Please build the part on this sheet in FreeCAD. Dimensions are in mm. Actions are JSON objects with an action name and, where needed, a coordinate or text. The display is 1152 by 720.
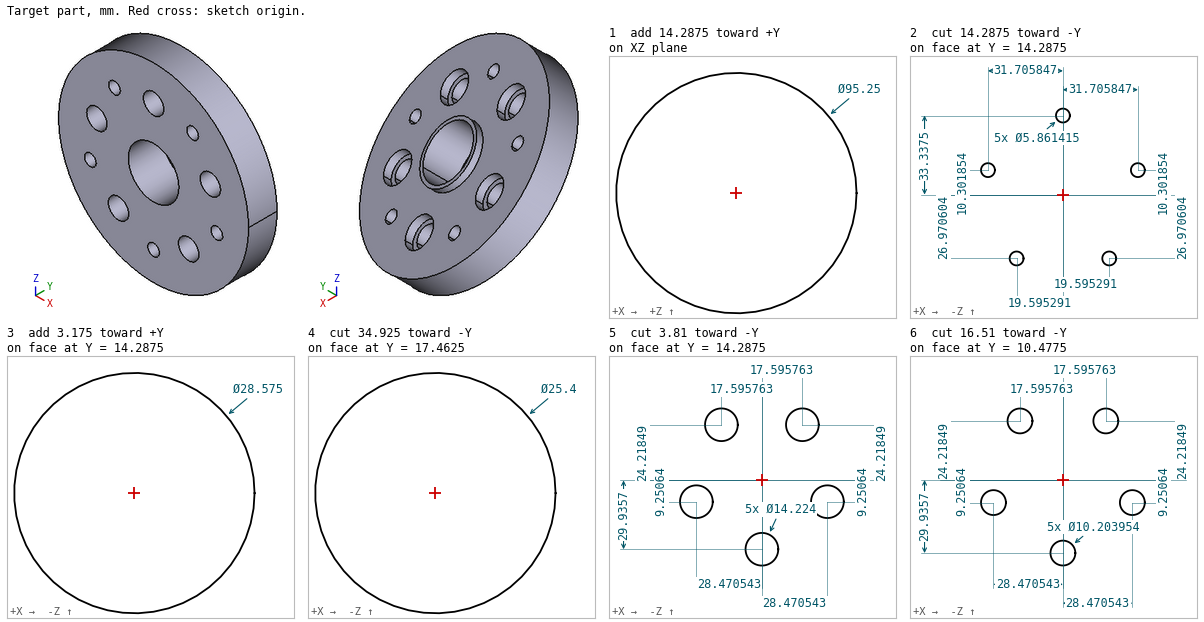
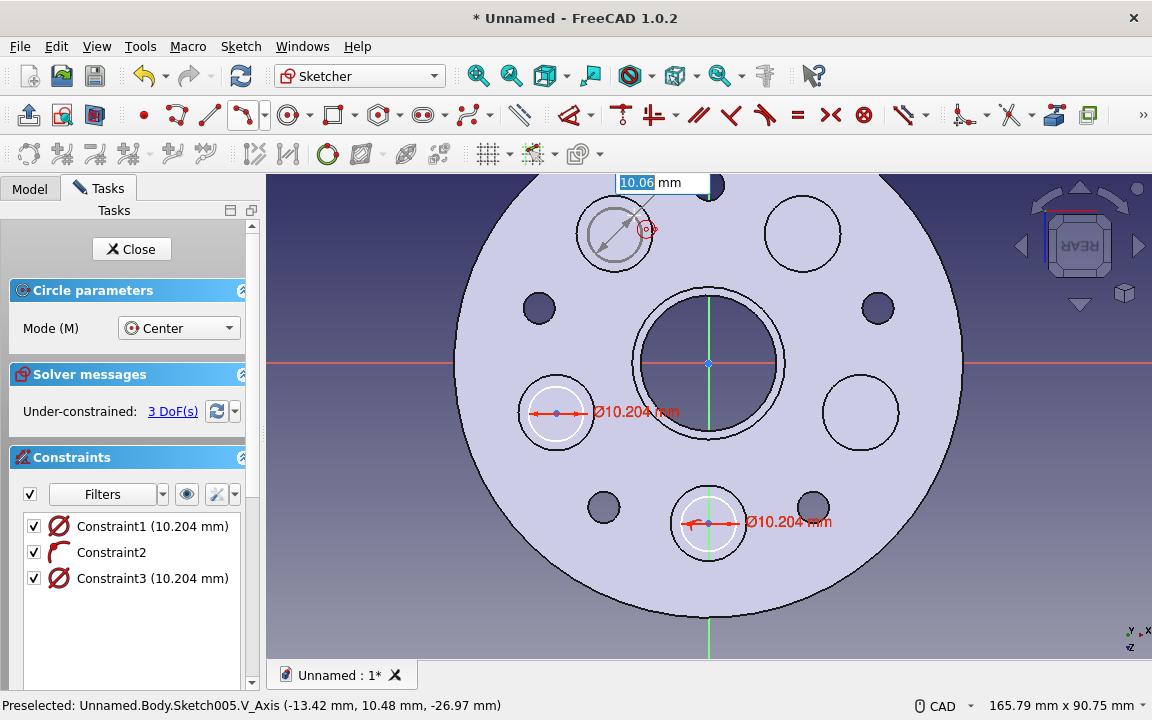
{"action": "type", "text": "10.203954"}
{"action": "key", "text": "Return"}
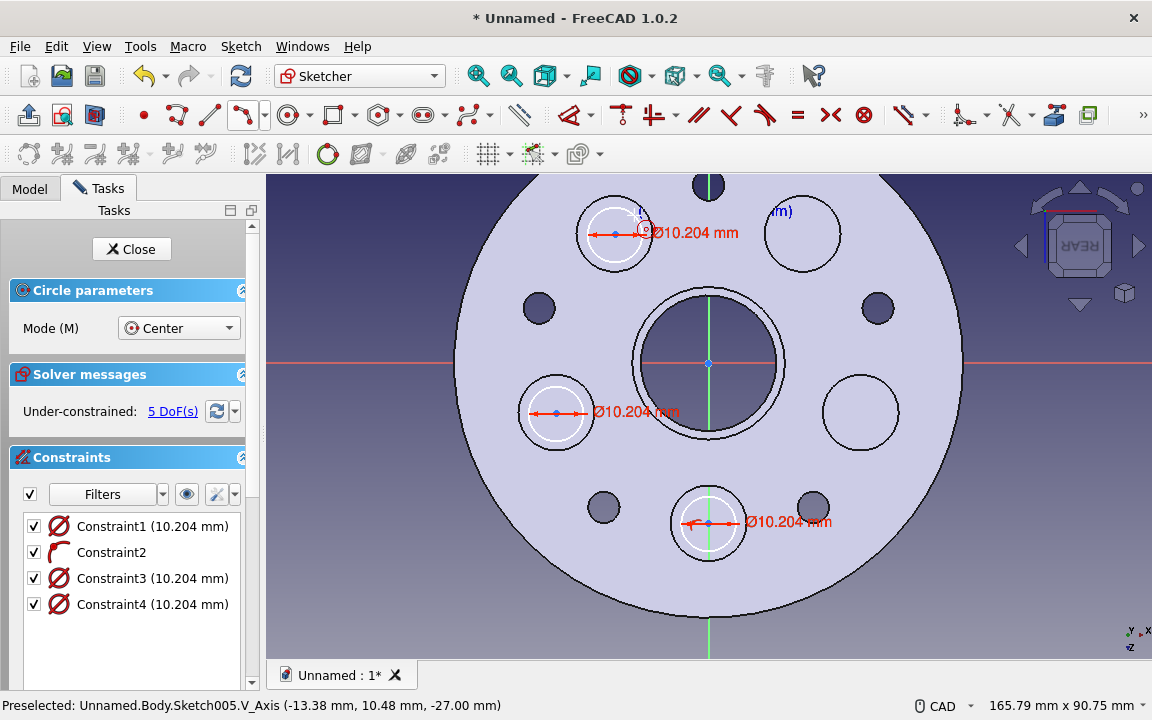
{"action": "left_click", "coordinate": [803, 234]}
{"action": "mouse_move", "coordinate": [822, 215]}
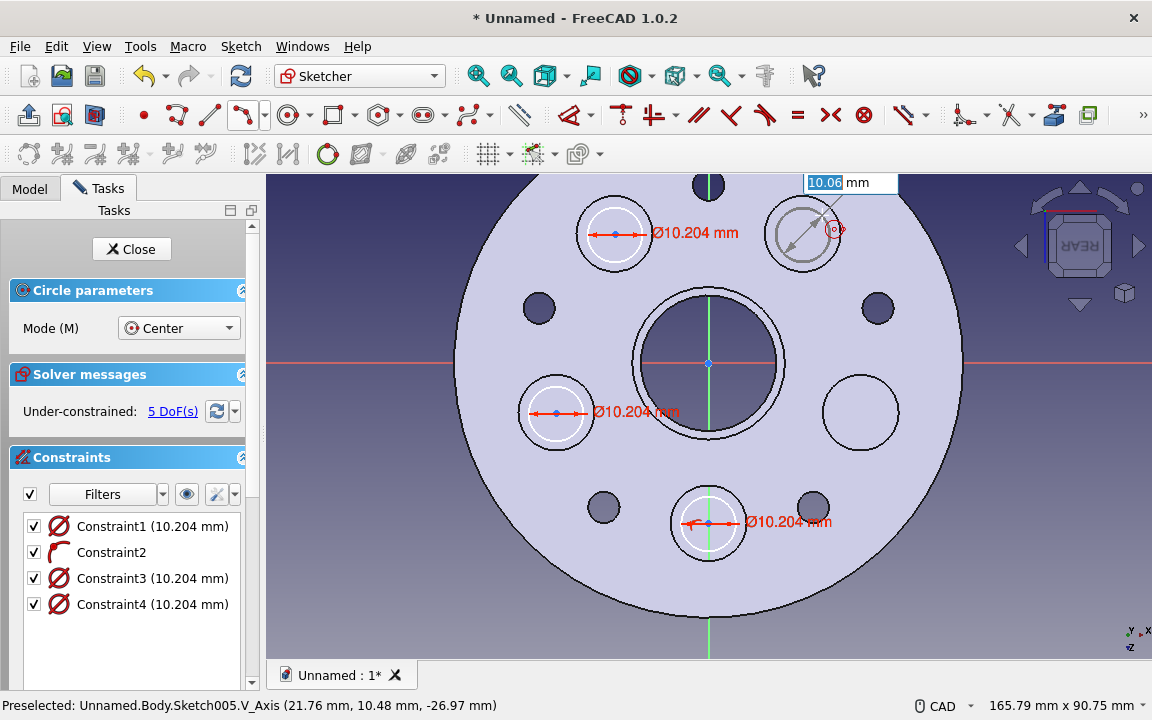
{"action": "type", "text": "10.203954"}
{"action": "key", "text": "Return"}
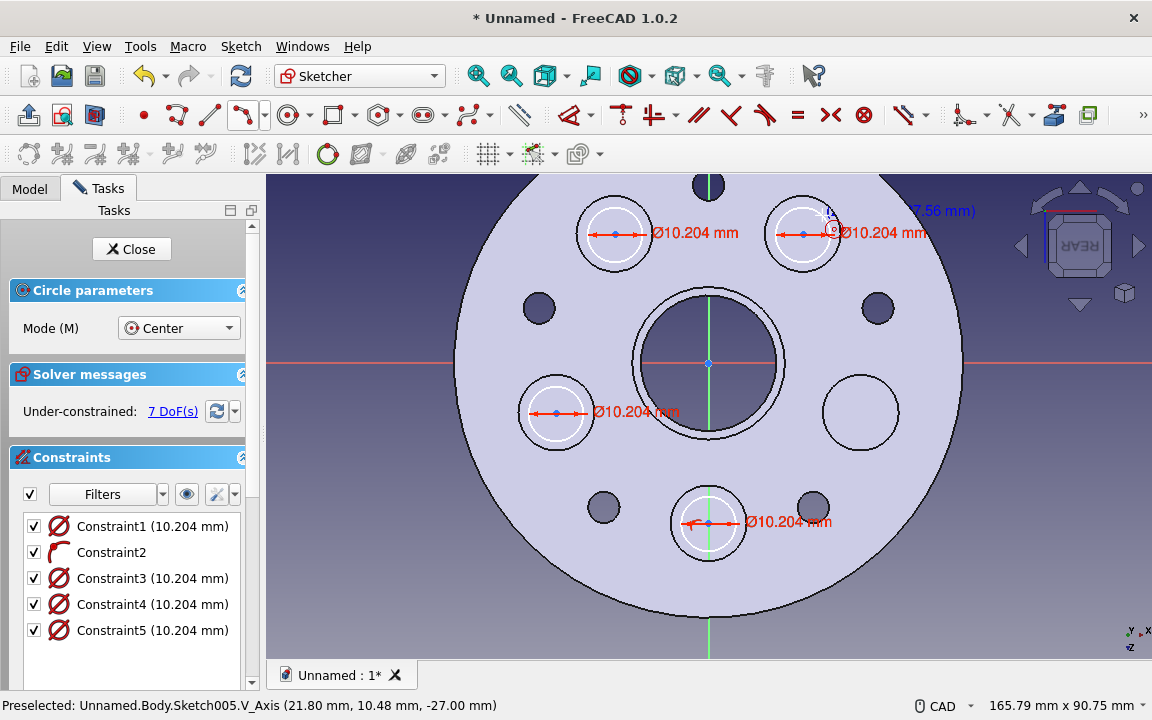
{"action": "left_click", "coordinate": [861, 413]}
{"action": "mouse_move", "coordinate": [880, 393]}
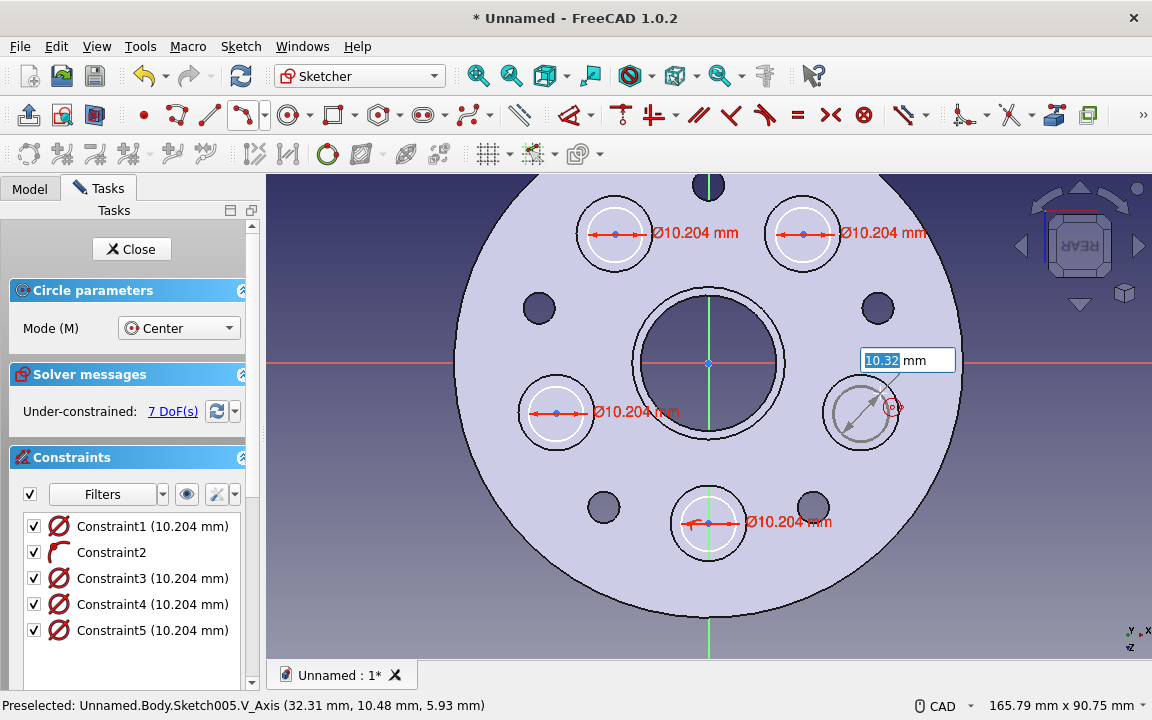
{"action": "type", "text": "10.203954"}
{"action": "key", "text": "Return"}
{"action": "key", "text": "Escape"}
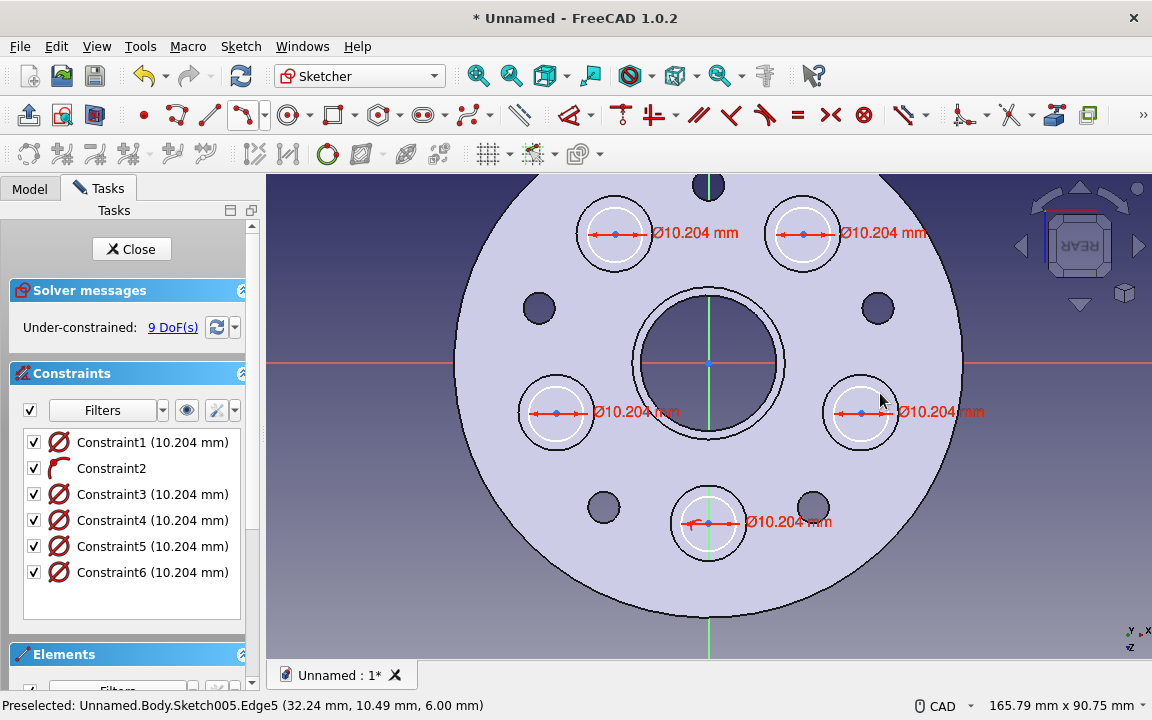
{"action": "left_click", "coordinate": [568, 116]}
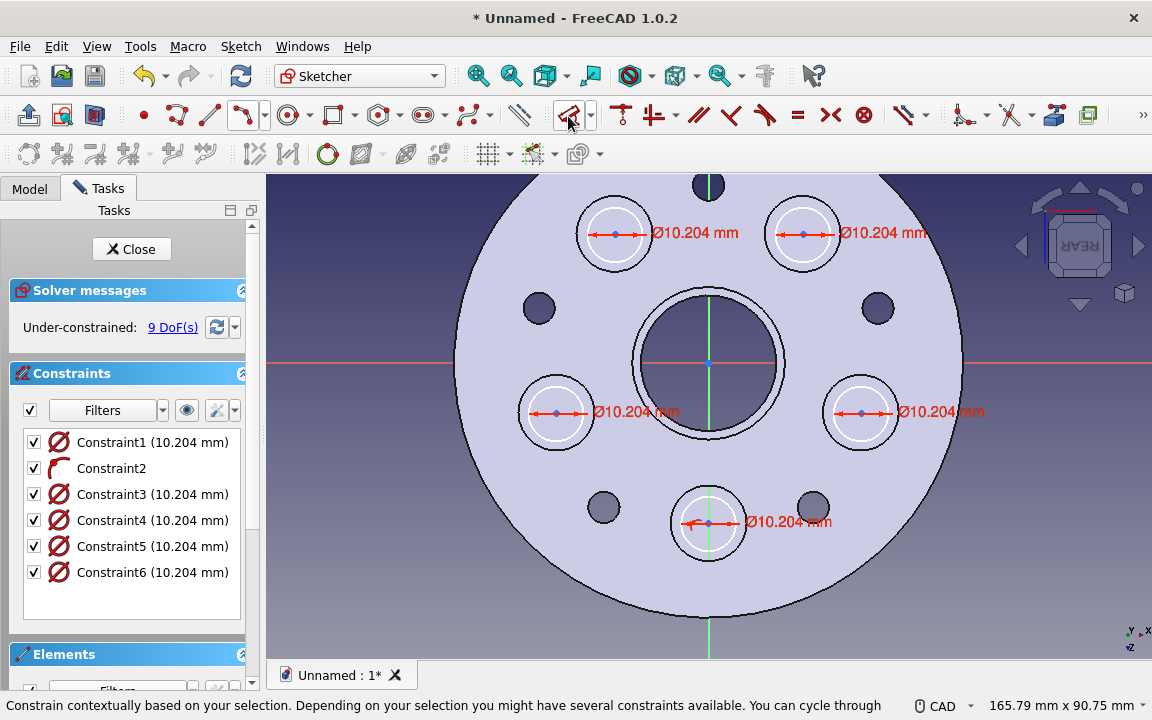
{"action": "left_click", "coordinate": [709, 524]}
{"action": "left_click", "coordinate": [743, 444]}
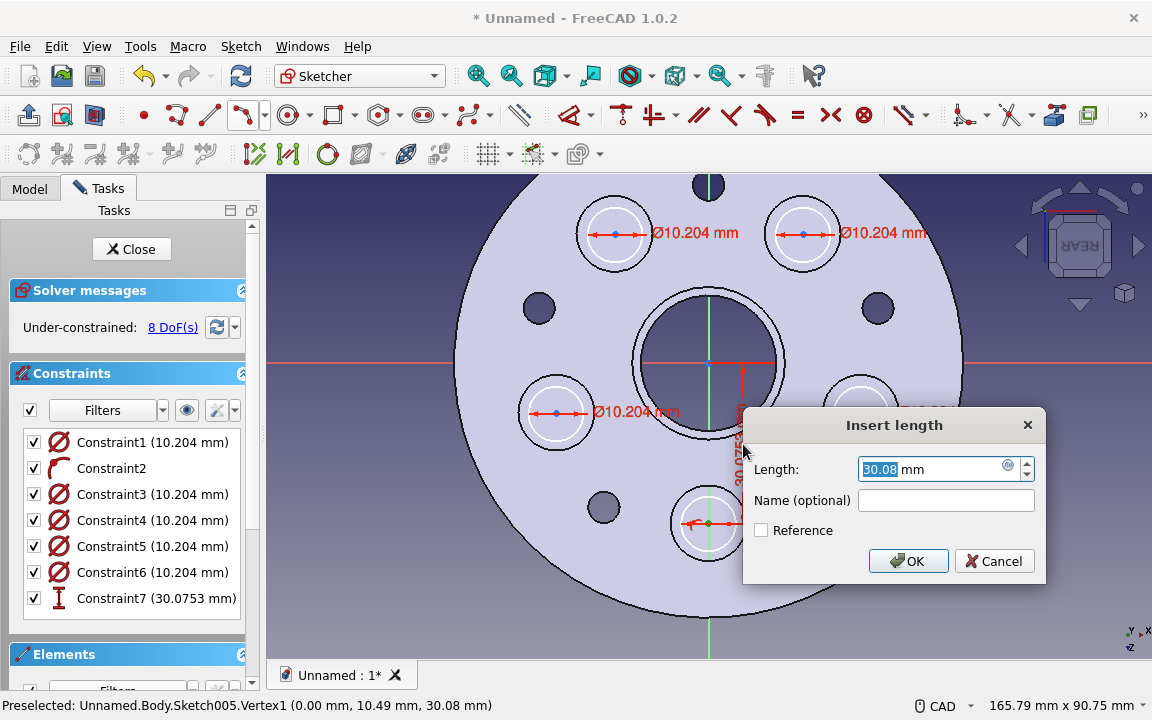
{"action": "type", "text": "29.9357"}
{"action": "key", "text": "Return"}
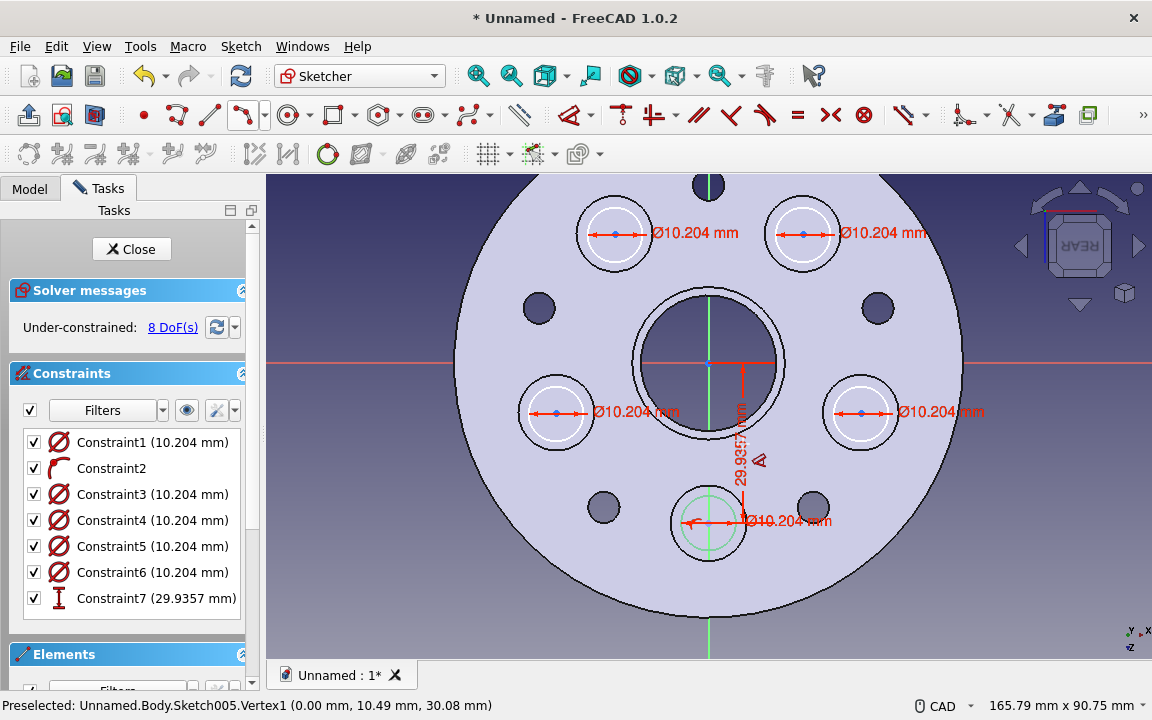
{"action": "left_click", "coordinate": [556, 414]}
{"action": "left_click", "coordinate": [522, 389]}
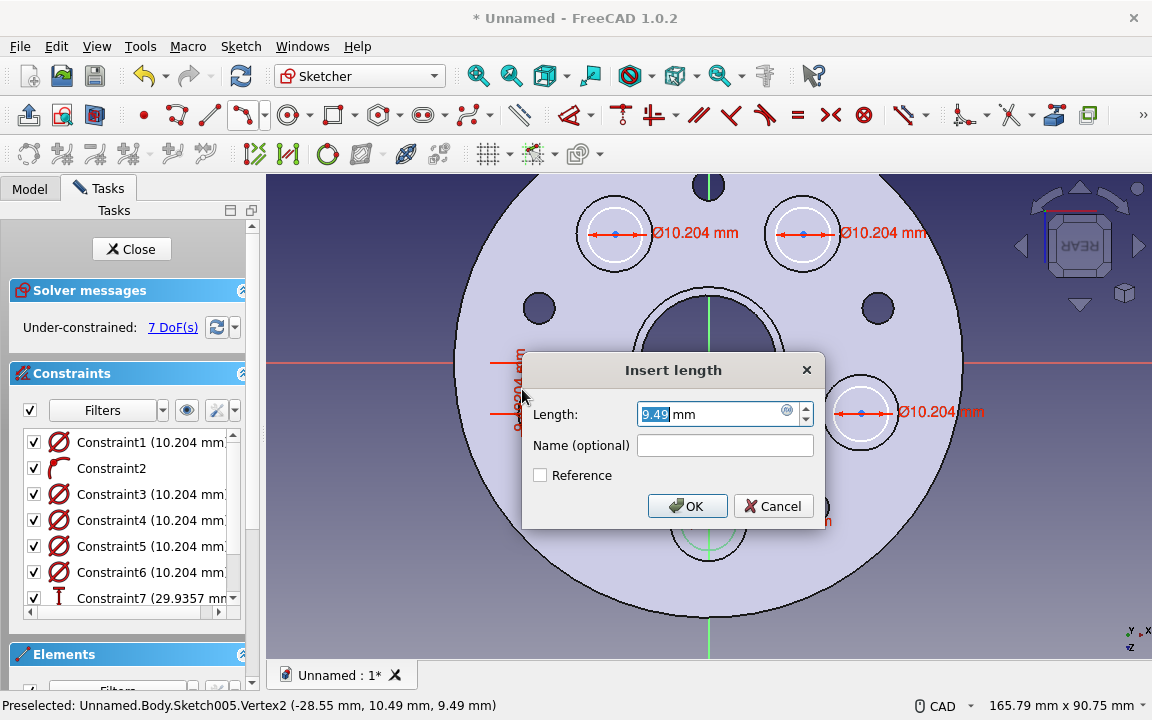
{"action": "type", "text": "9.25064"}
{"action": "key", "text": "Return"}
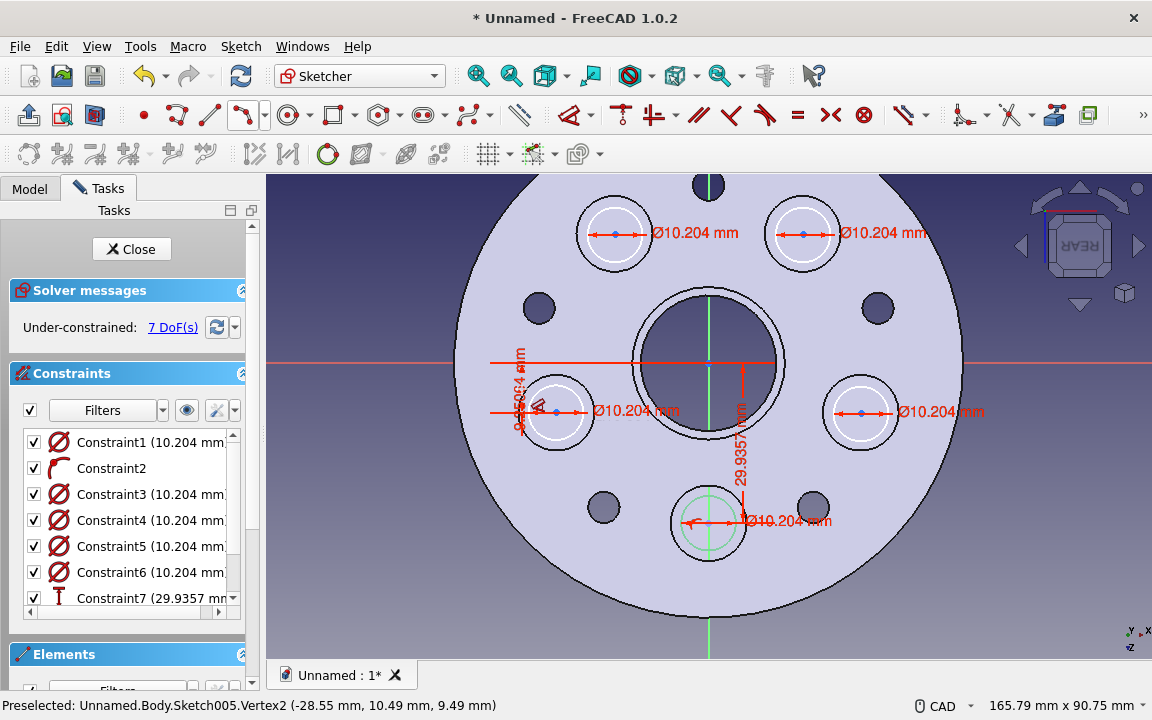
{"action": "left_click", "coordinate": [861, 414]}
{"action": "left_click", "coordinate": [895, 389]}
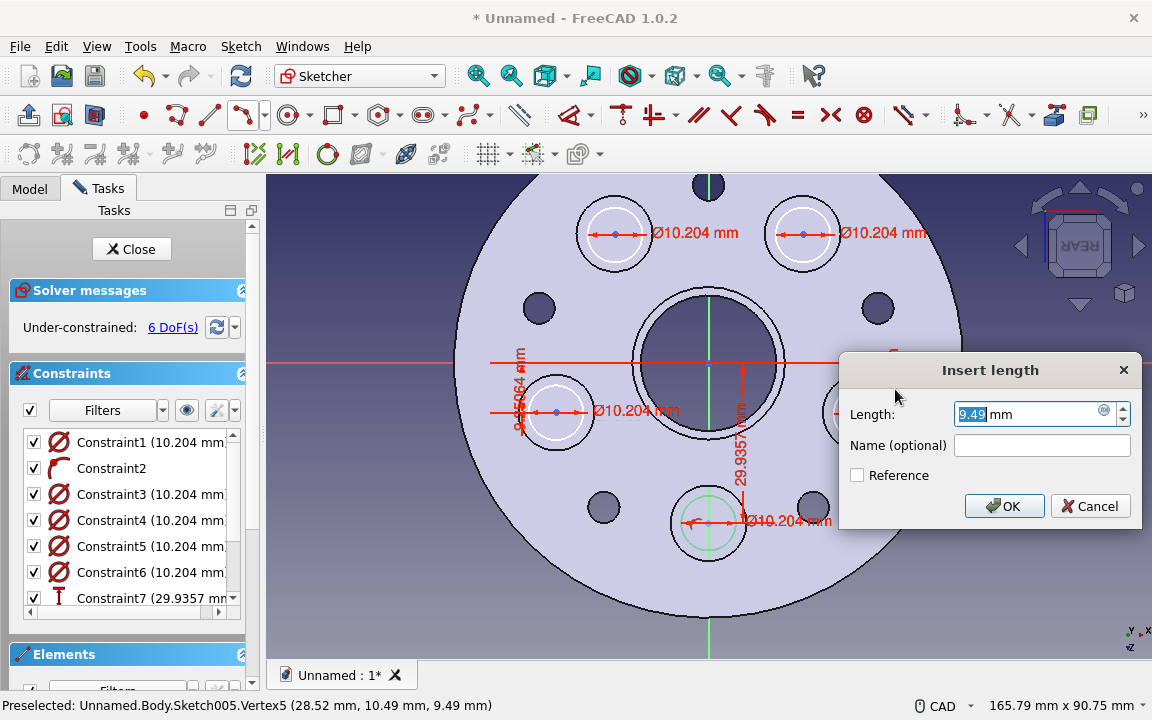
{"action": "type", "text": "9.25064"}
{"action": "key", "text": "Return"}